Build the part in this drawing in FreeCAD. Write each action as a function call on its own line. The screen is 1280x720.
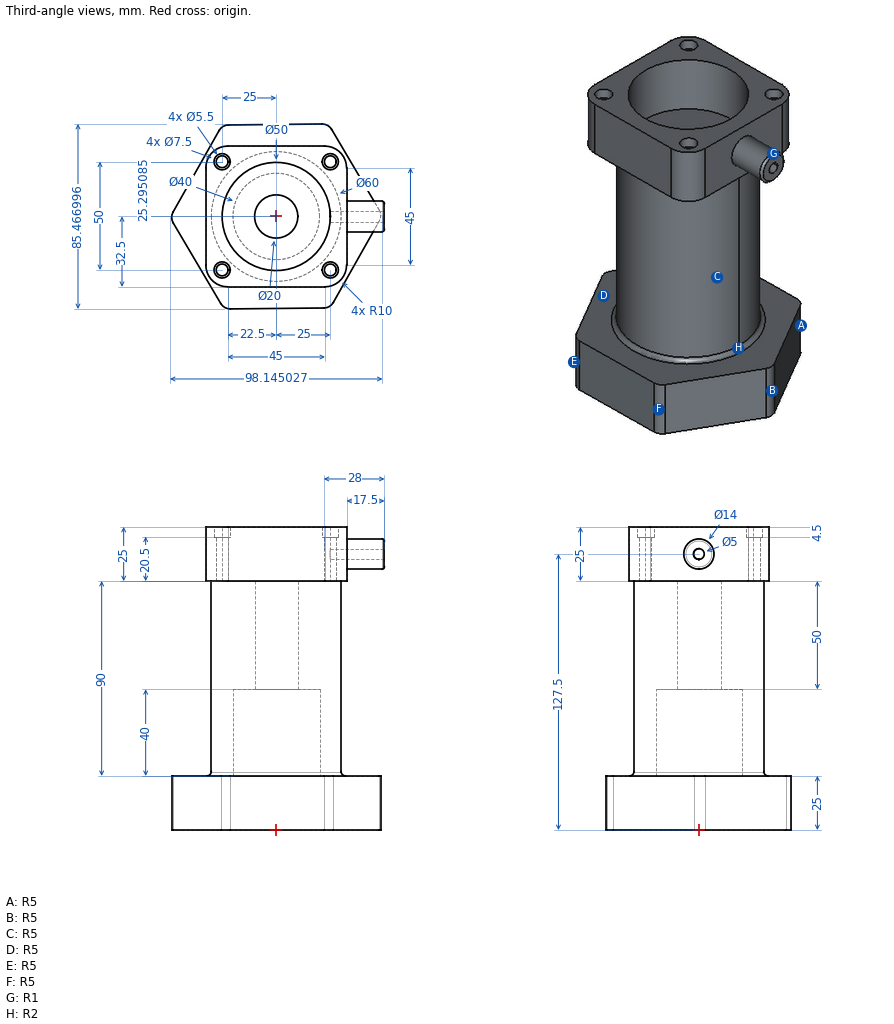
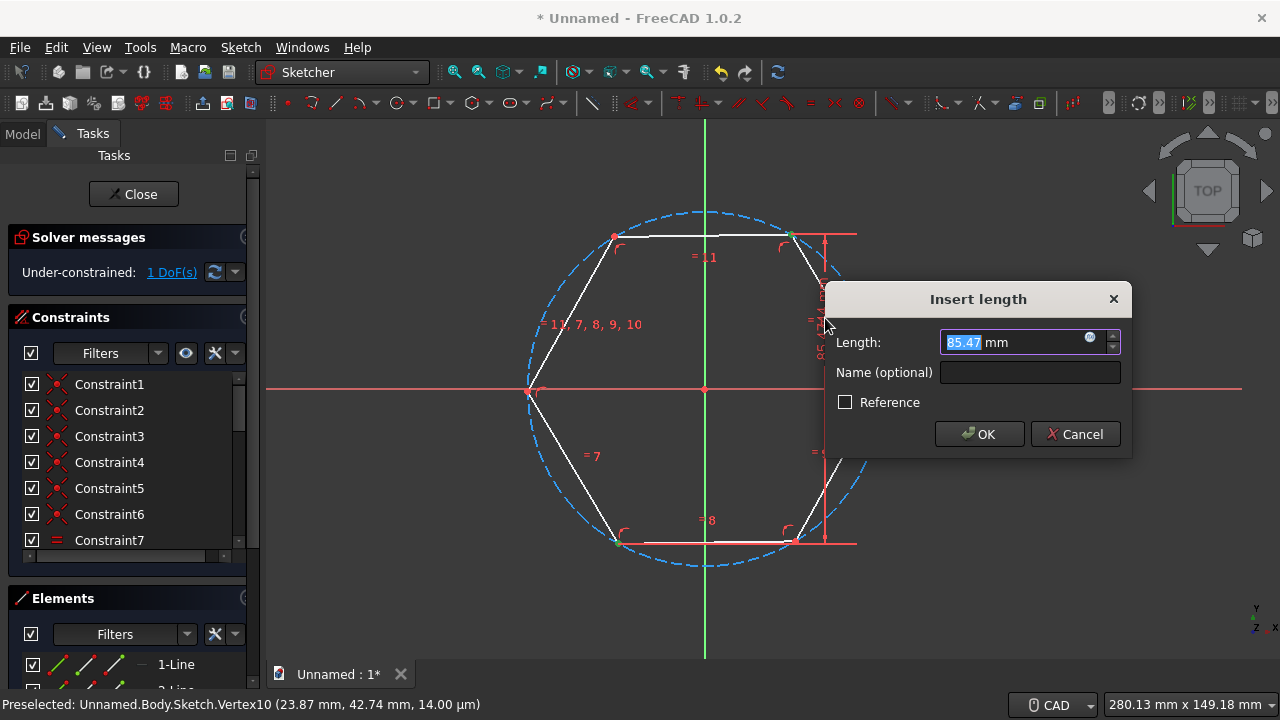
text(85.466996)
key(Return)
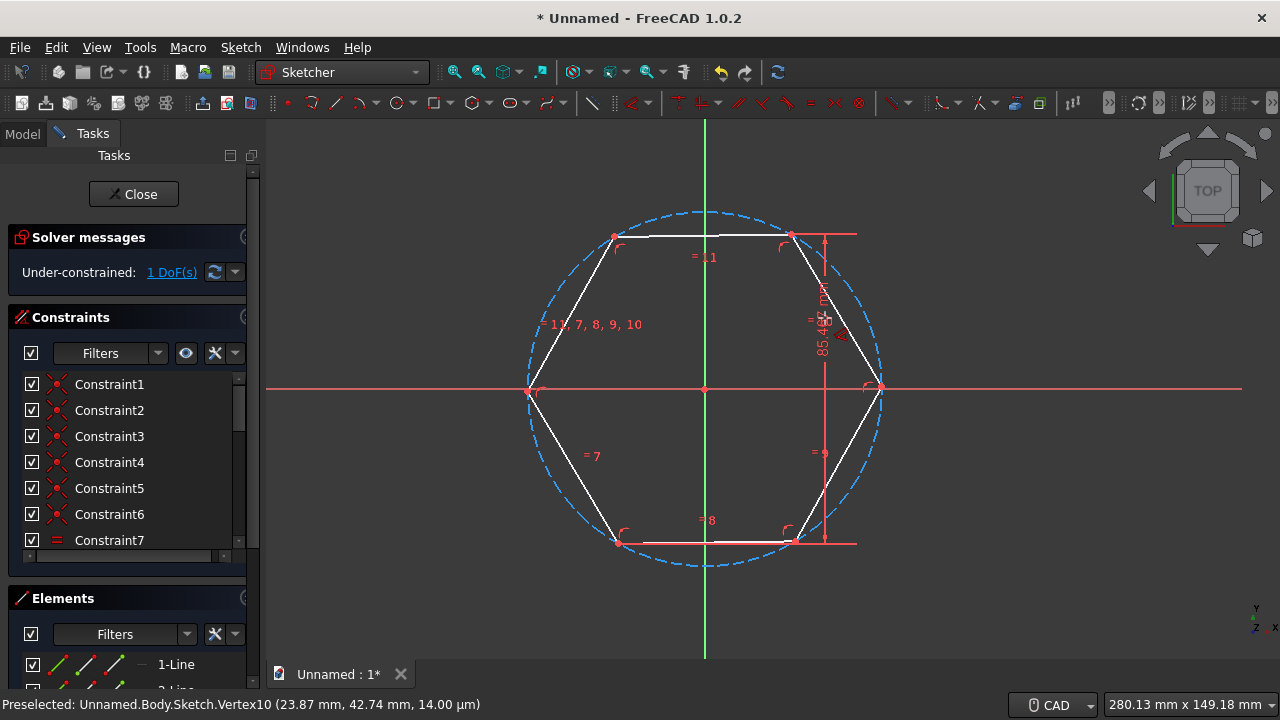
click(528, 392)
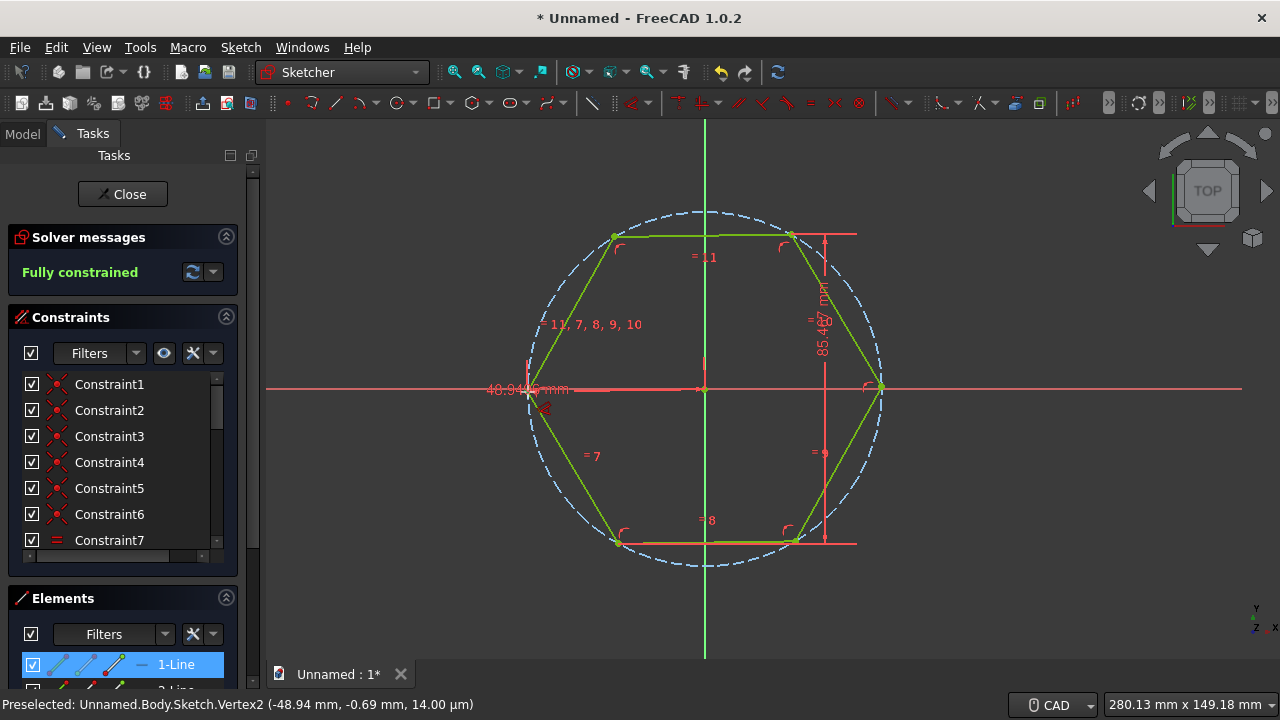
click(882, 387)
click(623, 353)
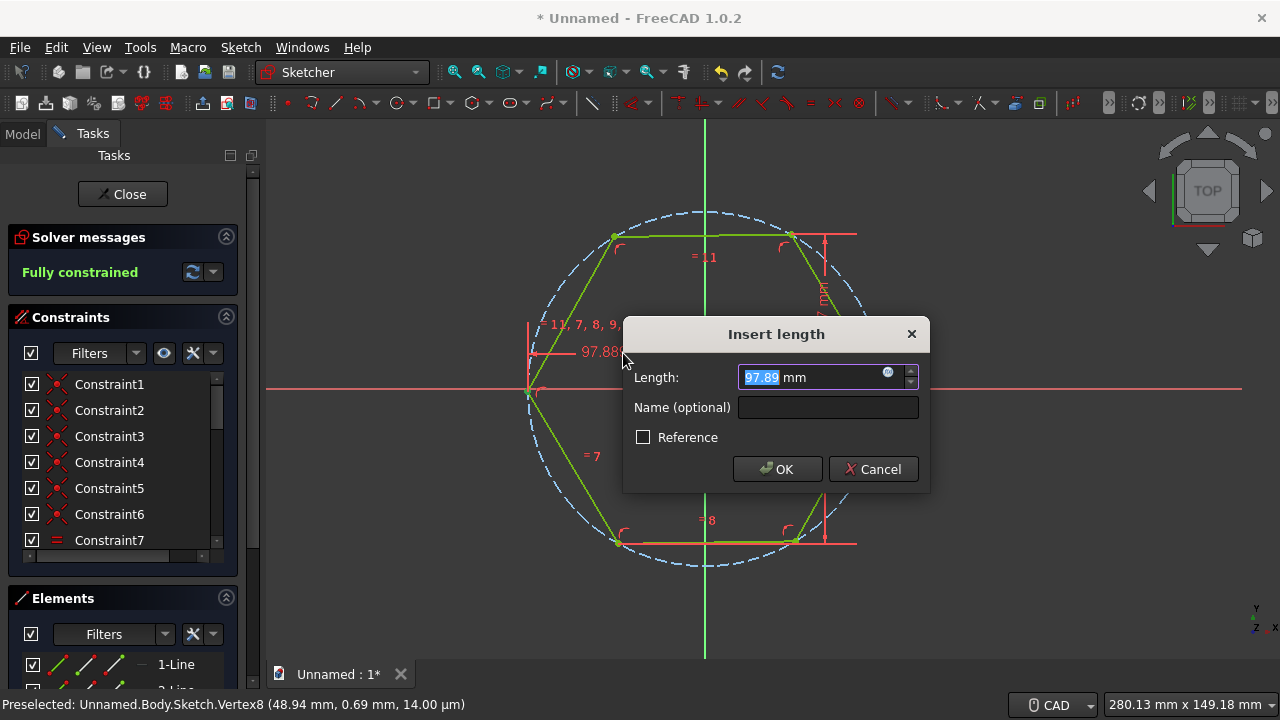
text(98.145027)
key(Return)
key(Escape)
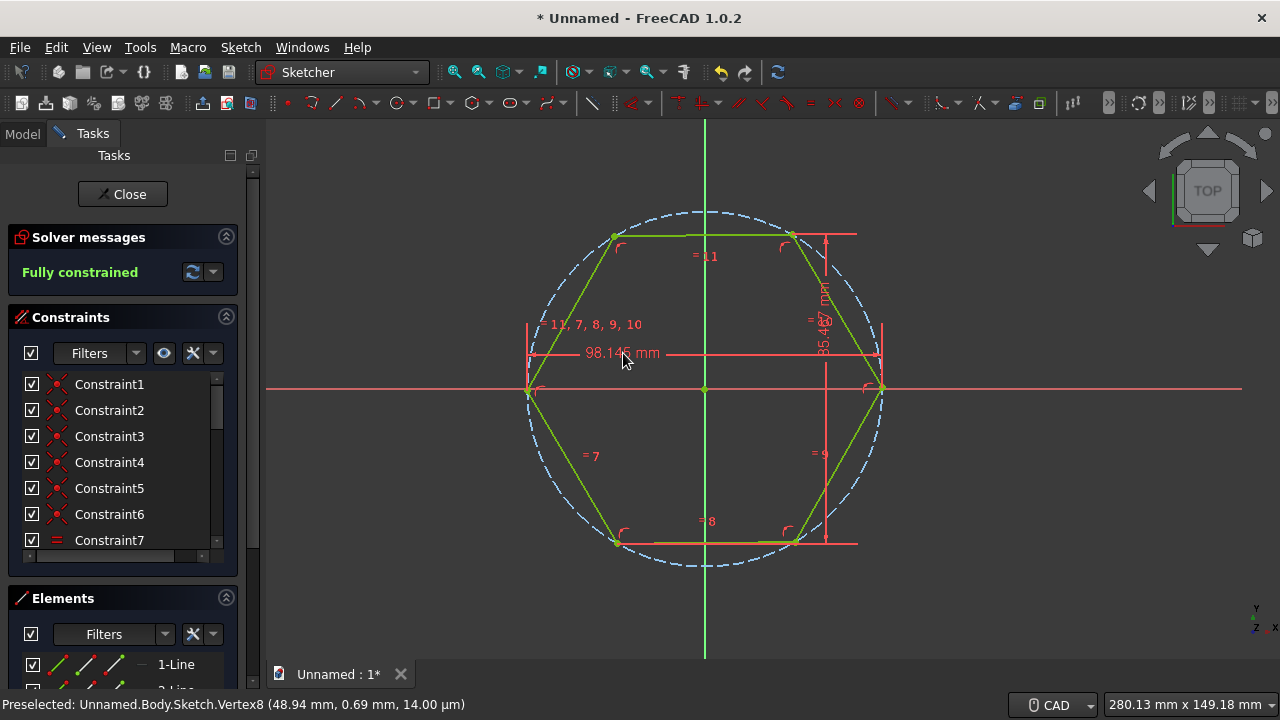
click(123, 194)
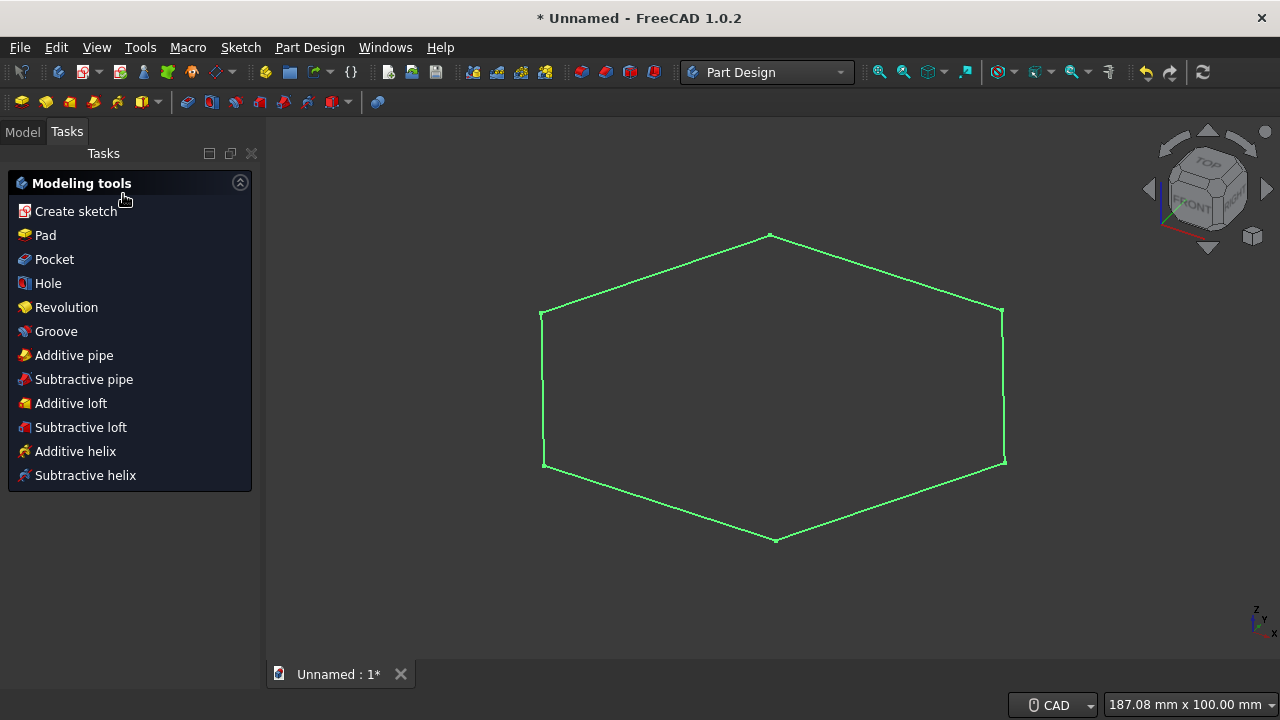
click(22, 102)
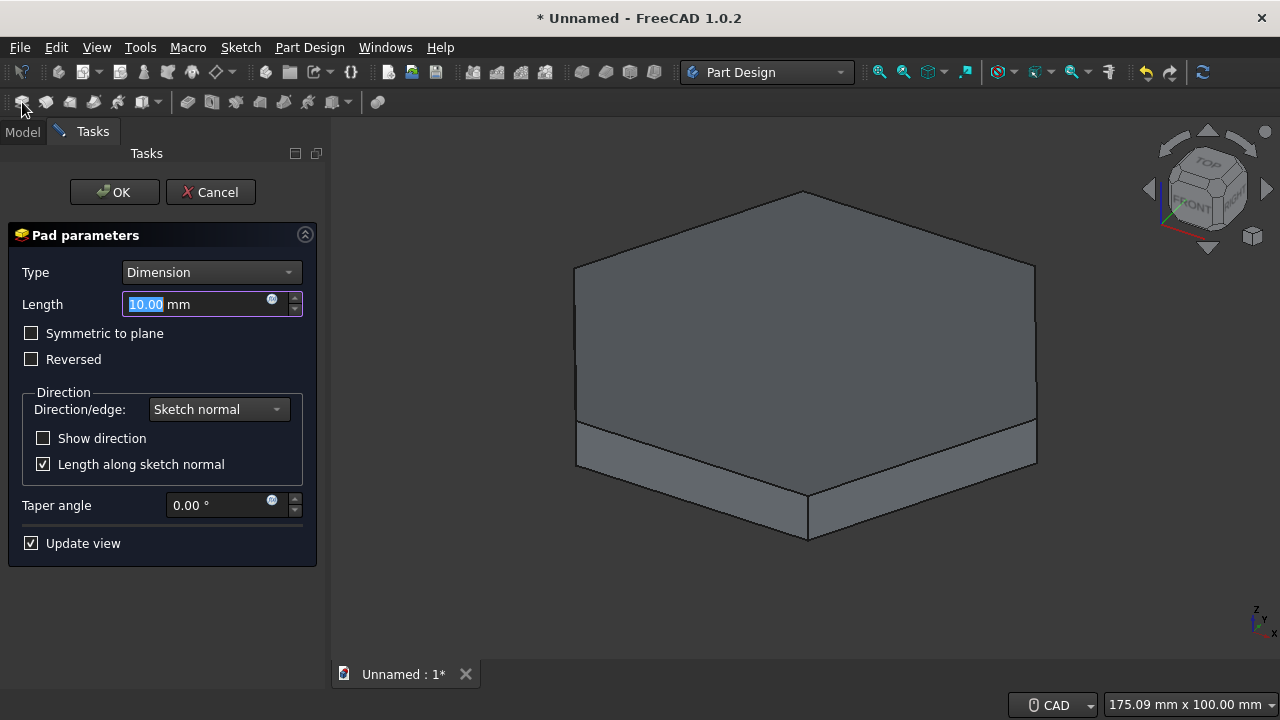
text(25)
key(Tab)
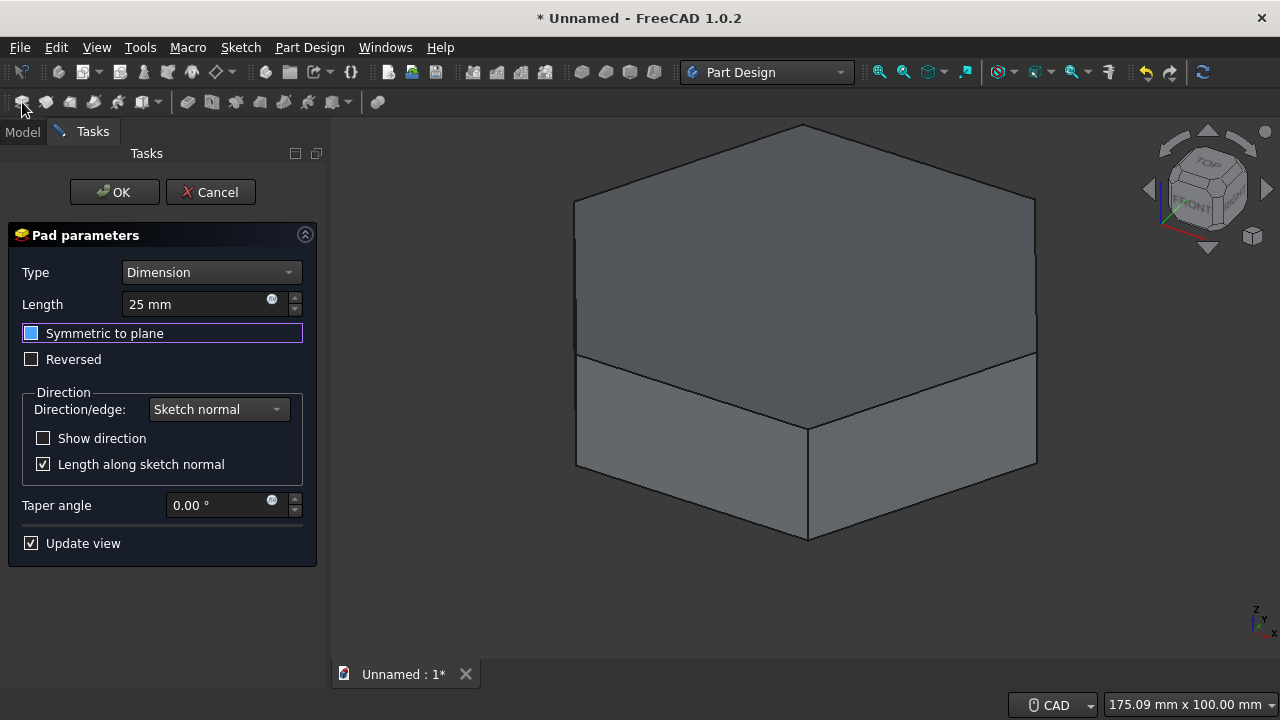
click(115, 192)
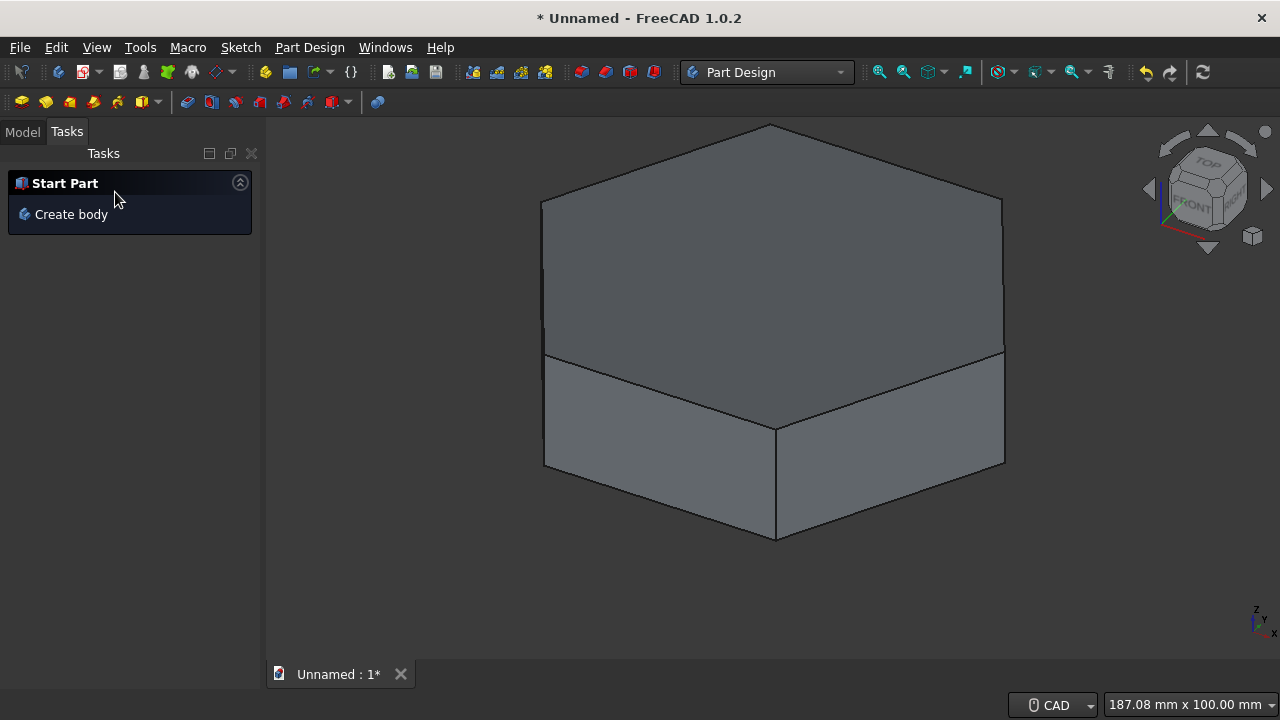
click(880, 72)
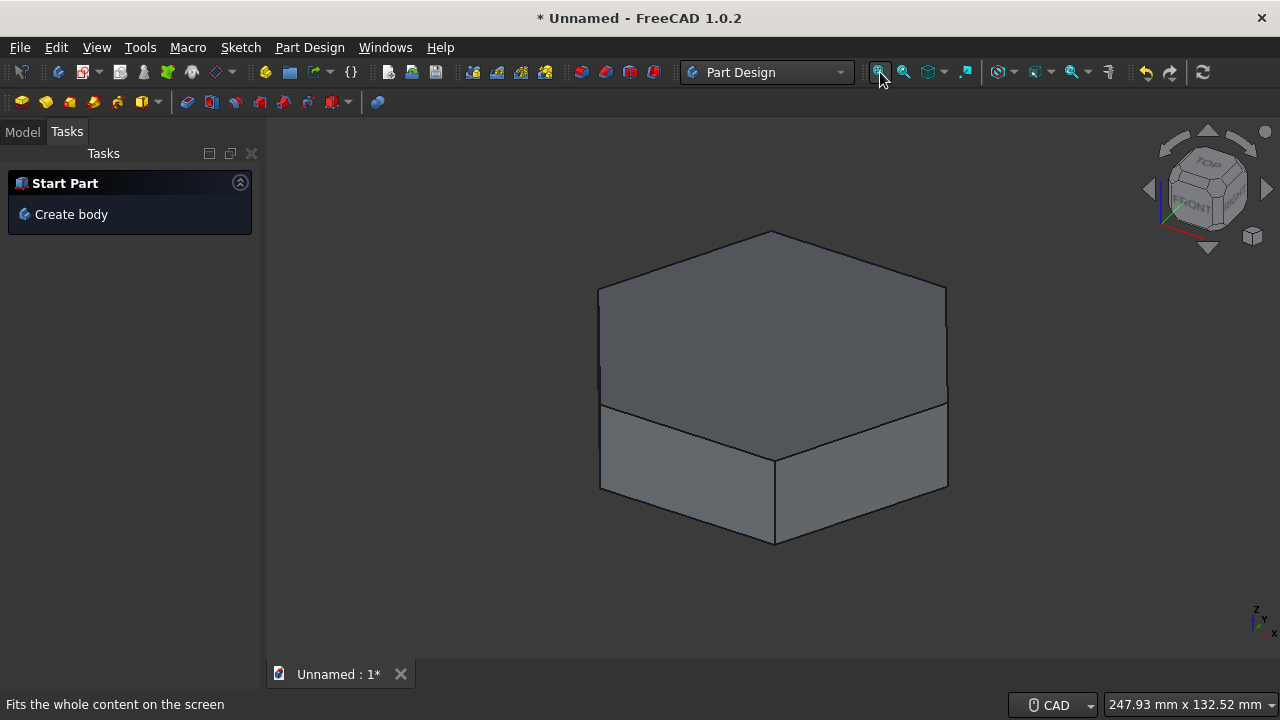
click(773, 345)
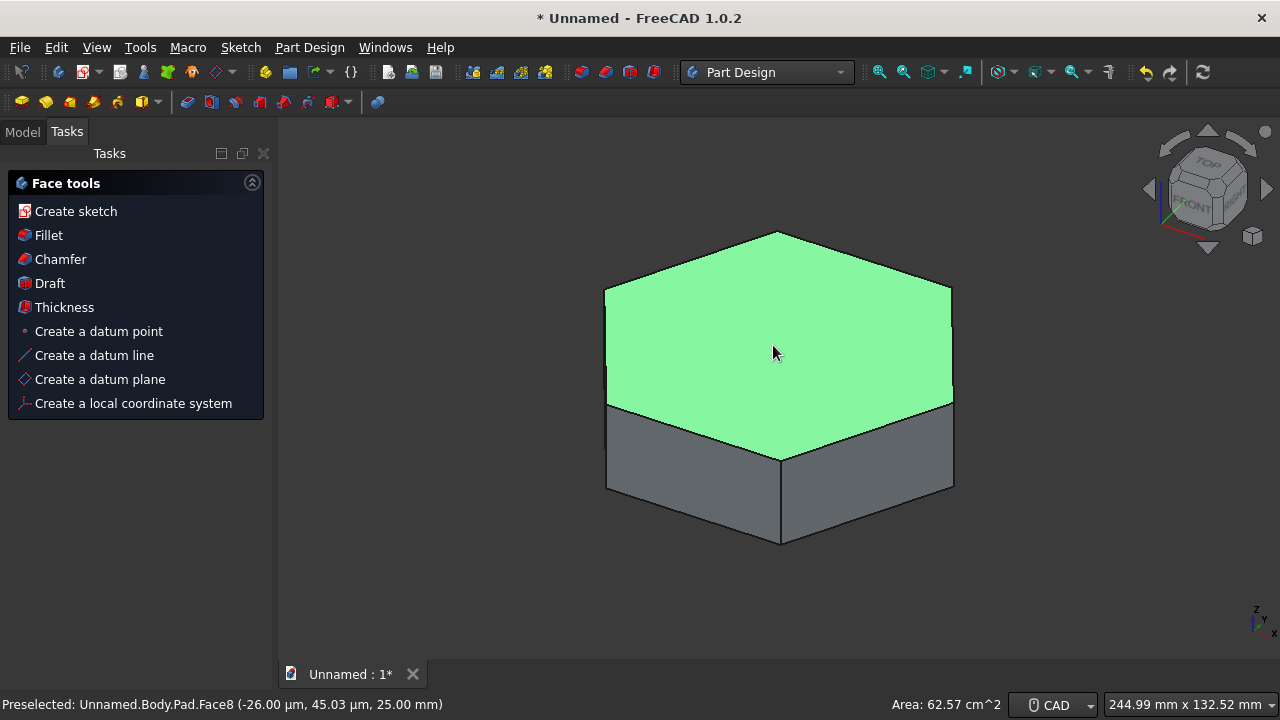
click(84, 72)